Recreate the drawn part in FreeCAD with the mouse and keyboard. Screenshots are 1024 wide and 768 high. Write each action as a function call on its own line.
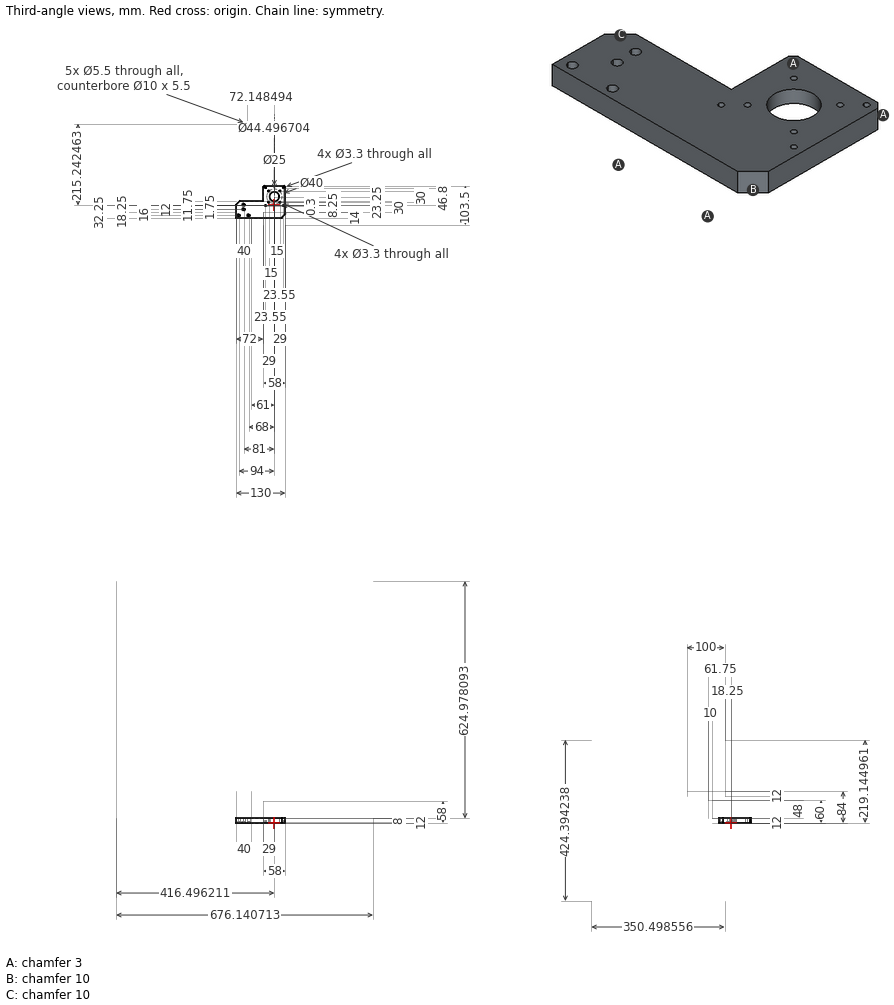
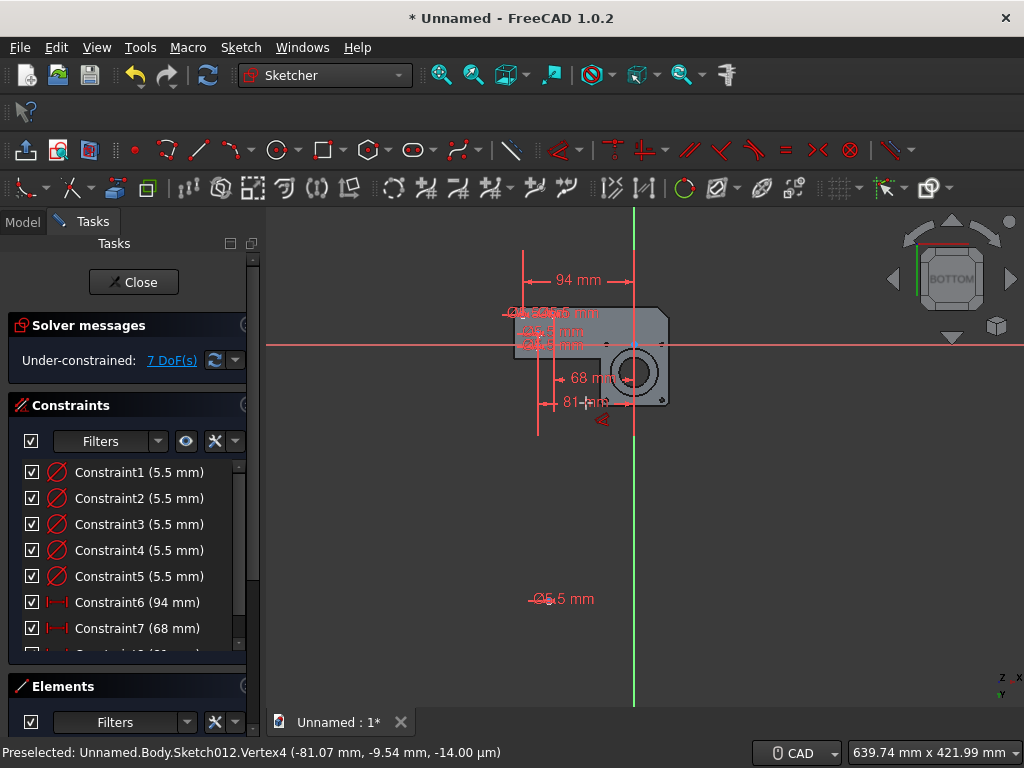
click(538, 347)
click(586, 311)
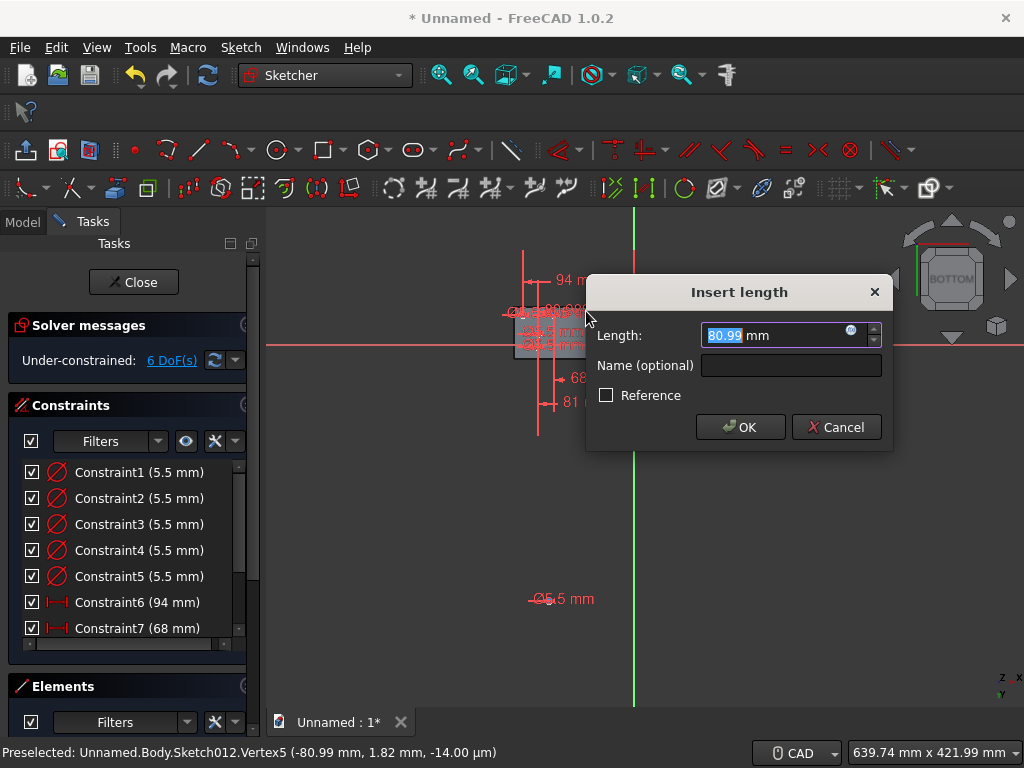
text(81)
key(Return)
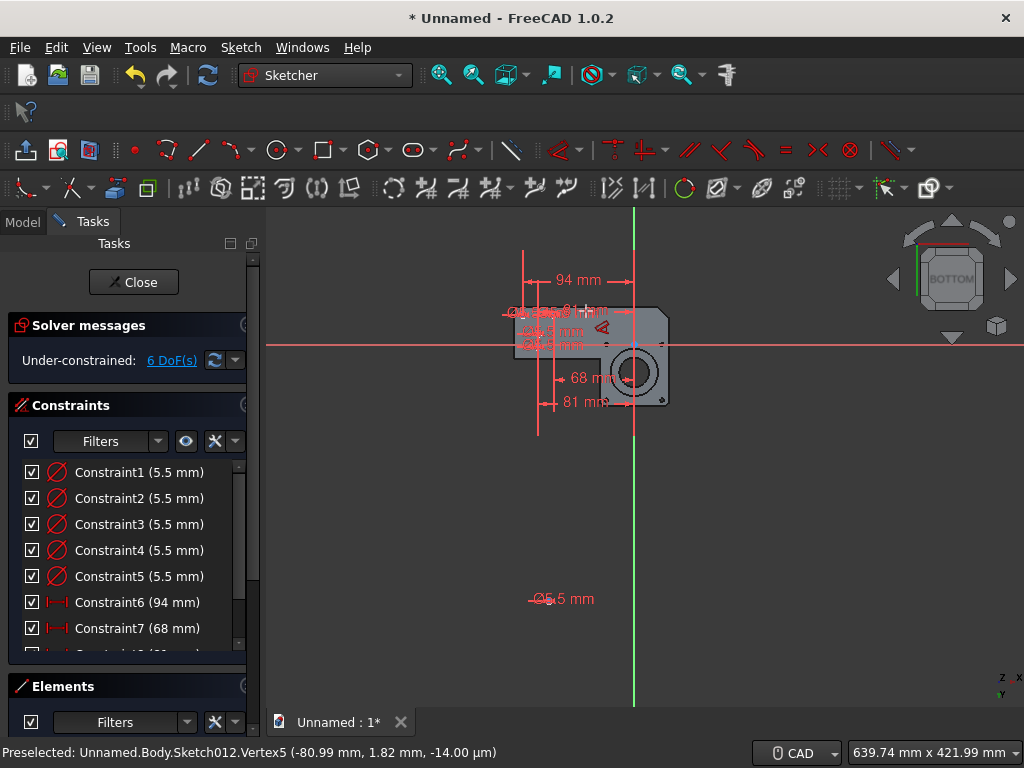
scroll(523, 315, up, 4)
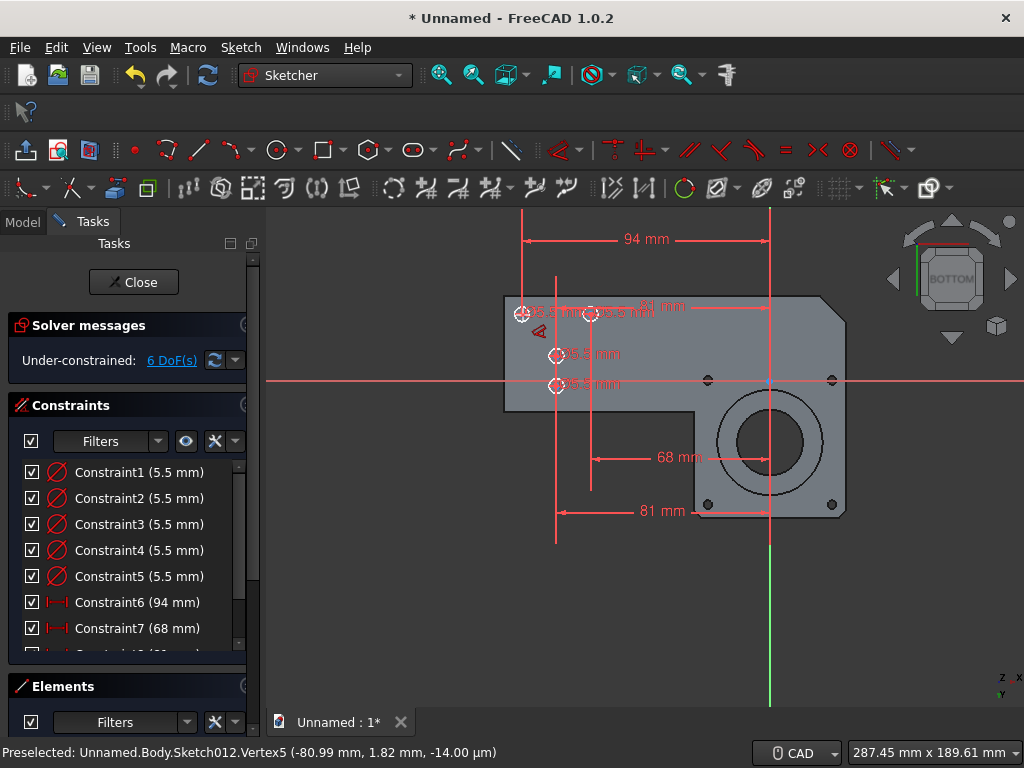
click(522, 314)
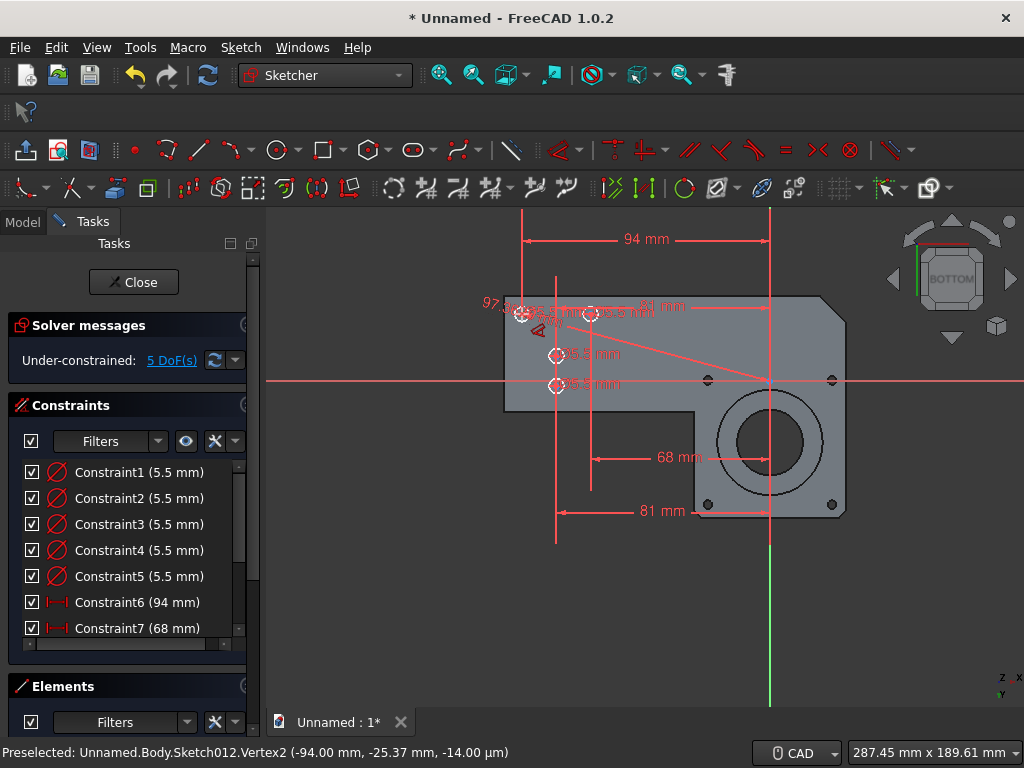
click(556, 356)
click(488, 335)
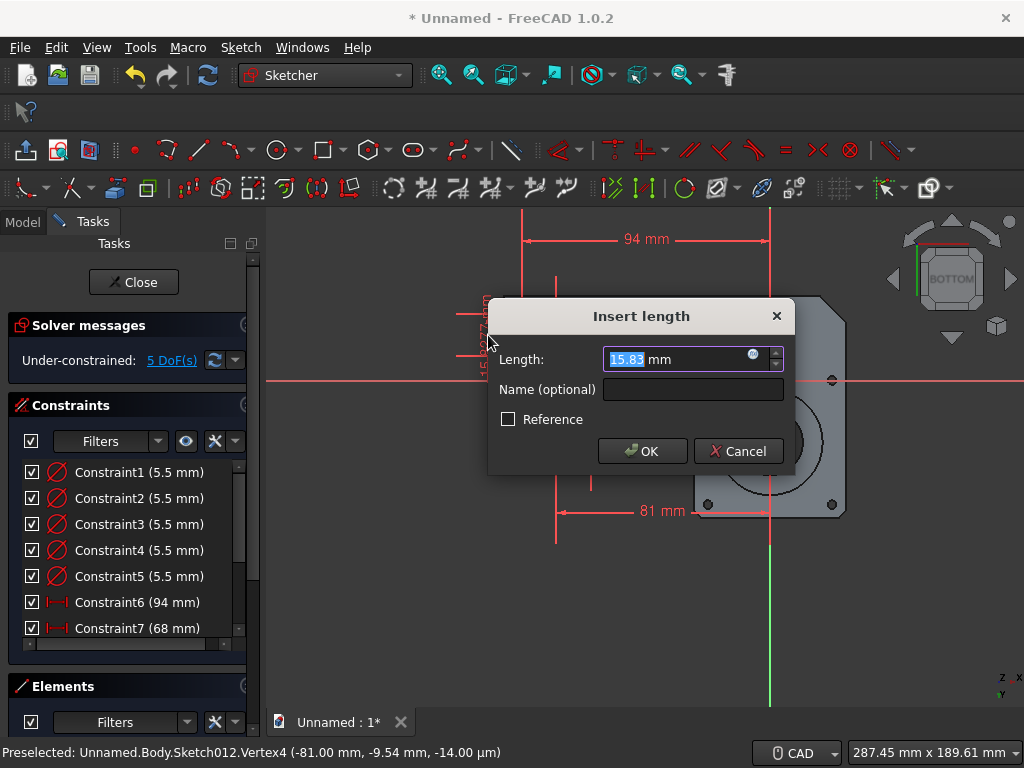
text(16)
key(Return)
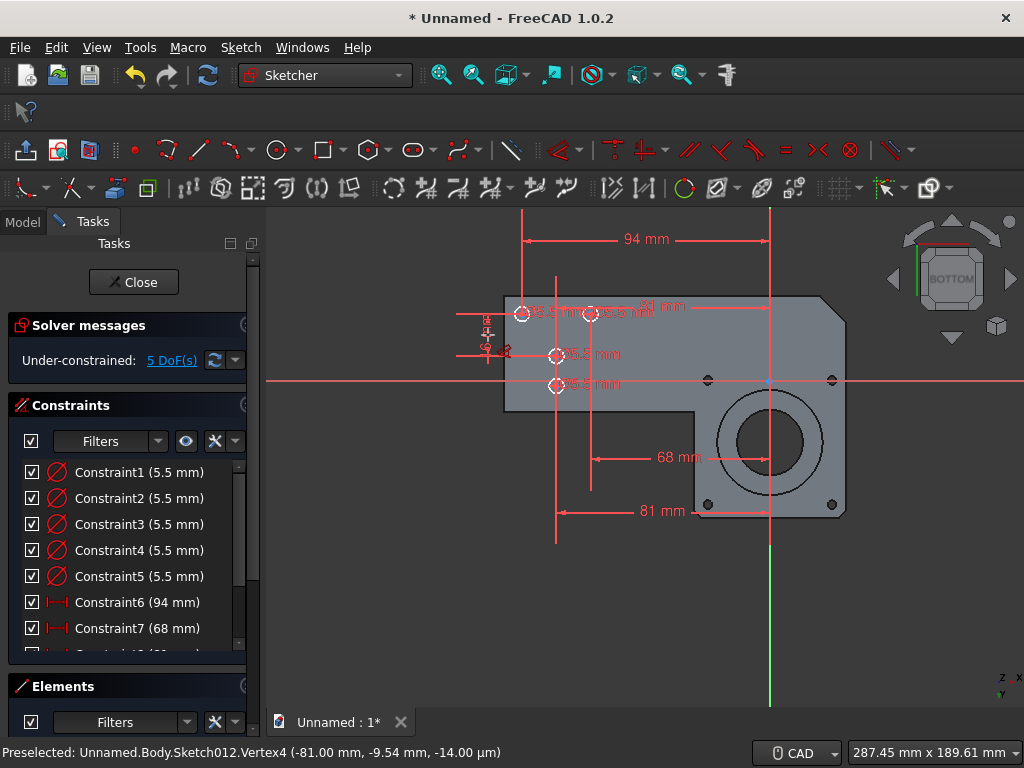
click(591, 314)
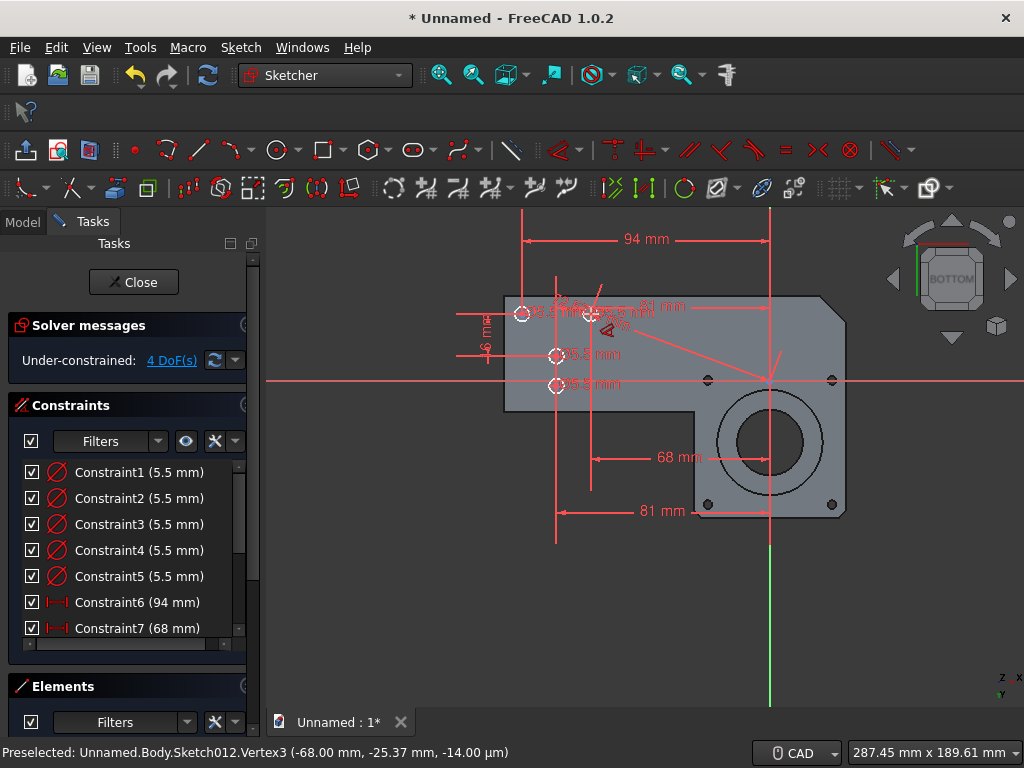
click(556, 356)
click(625, 335)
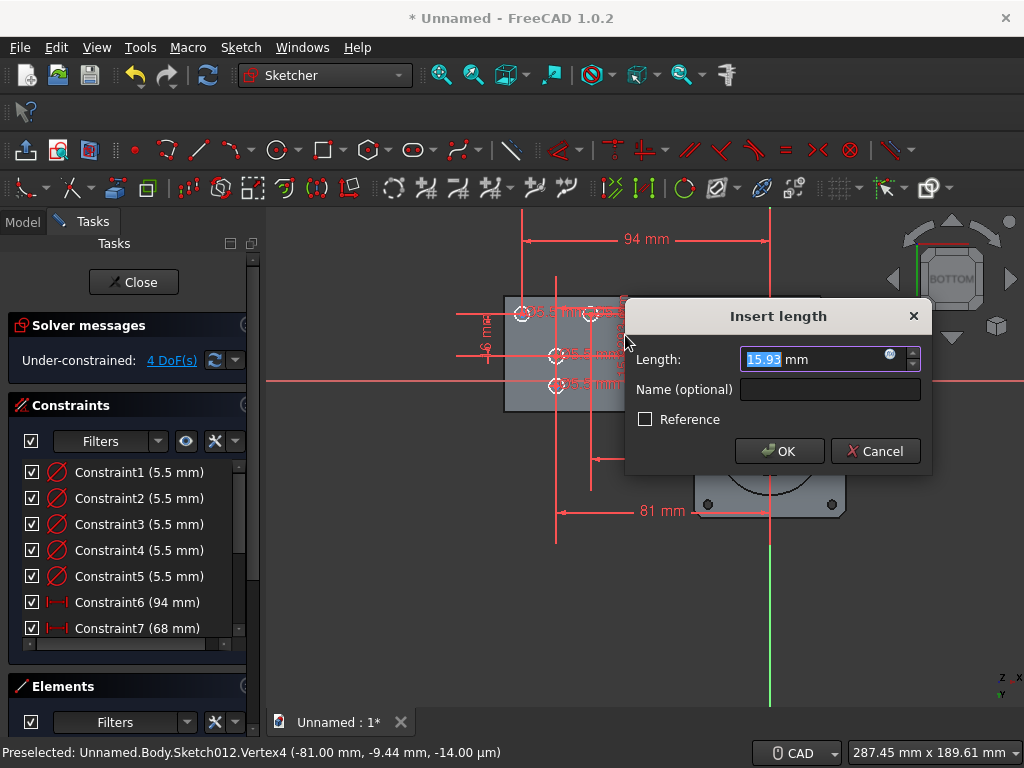
text(16)
key(Return)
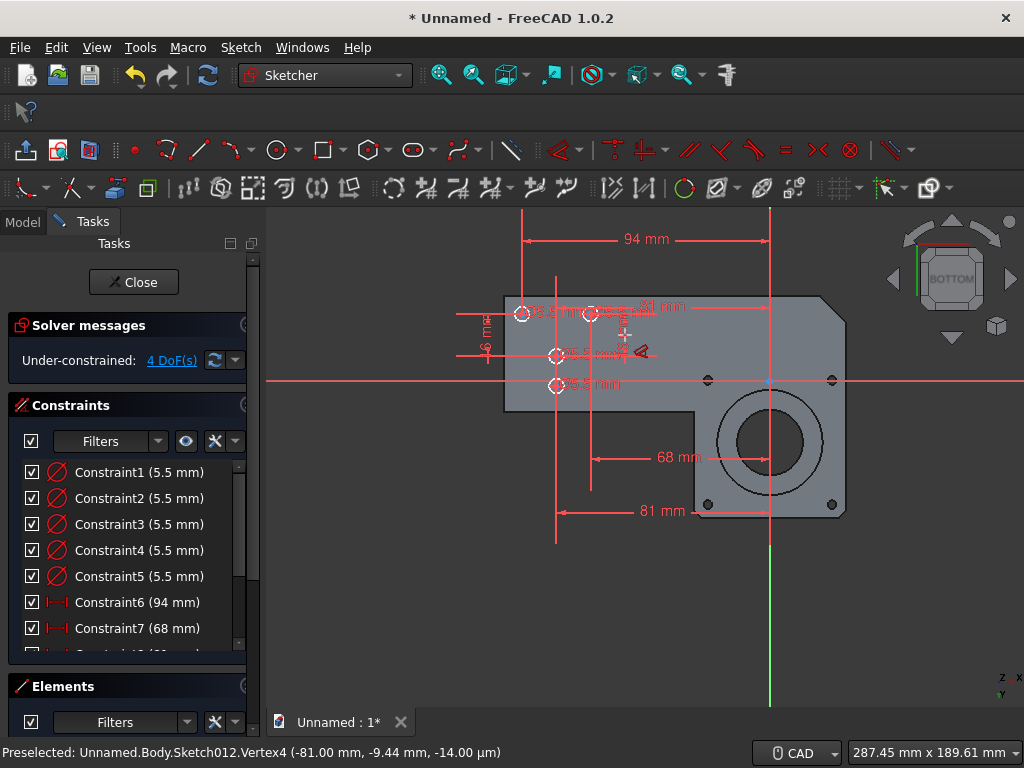
scroll(556, 356, up, 2)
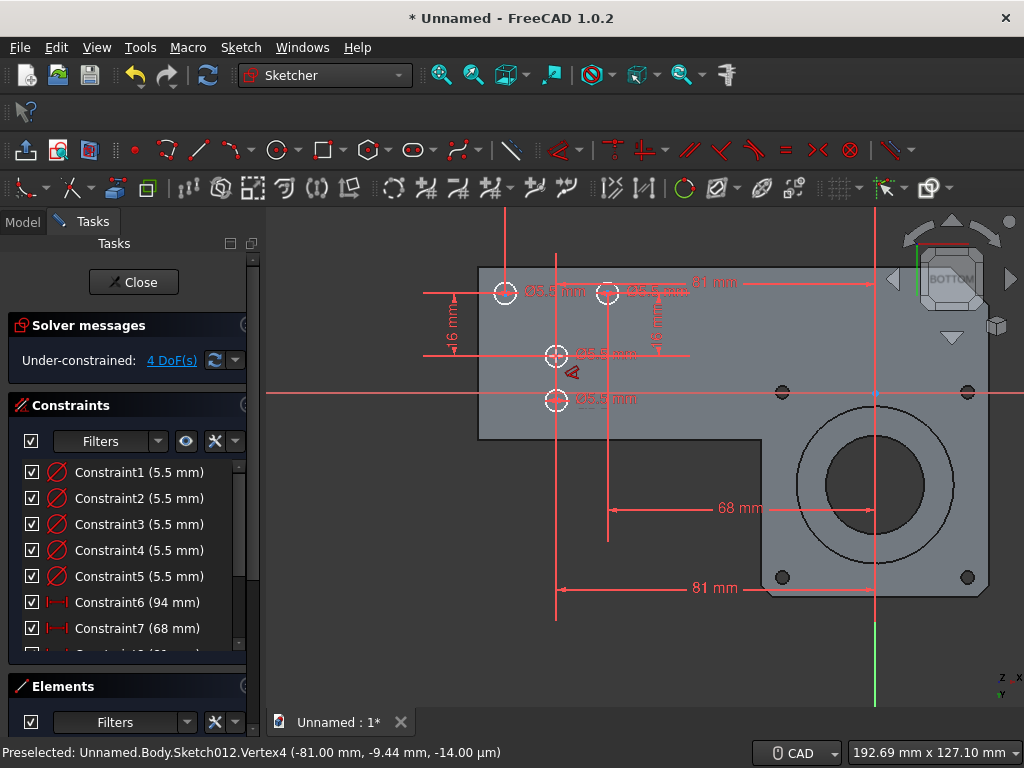
click(556, 356)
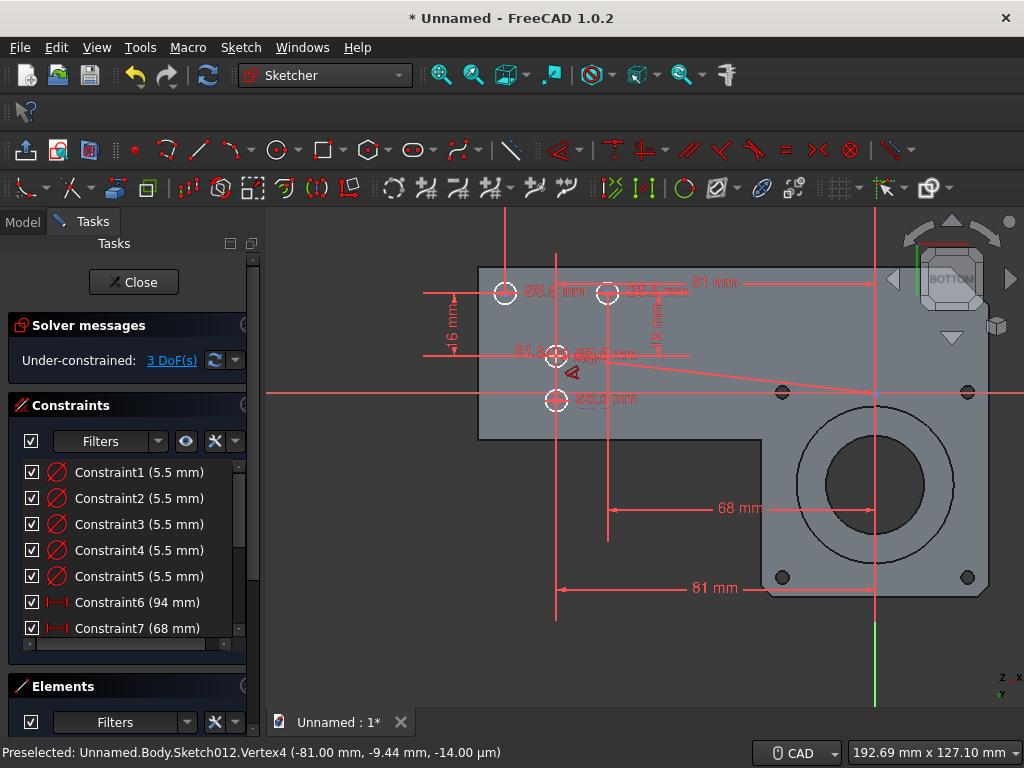
click(556, 401)
click(522, 378)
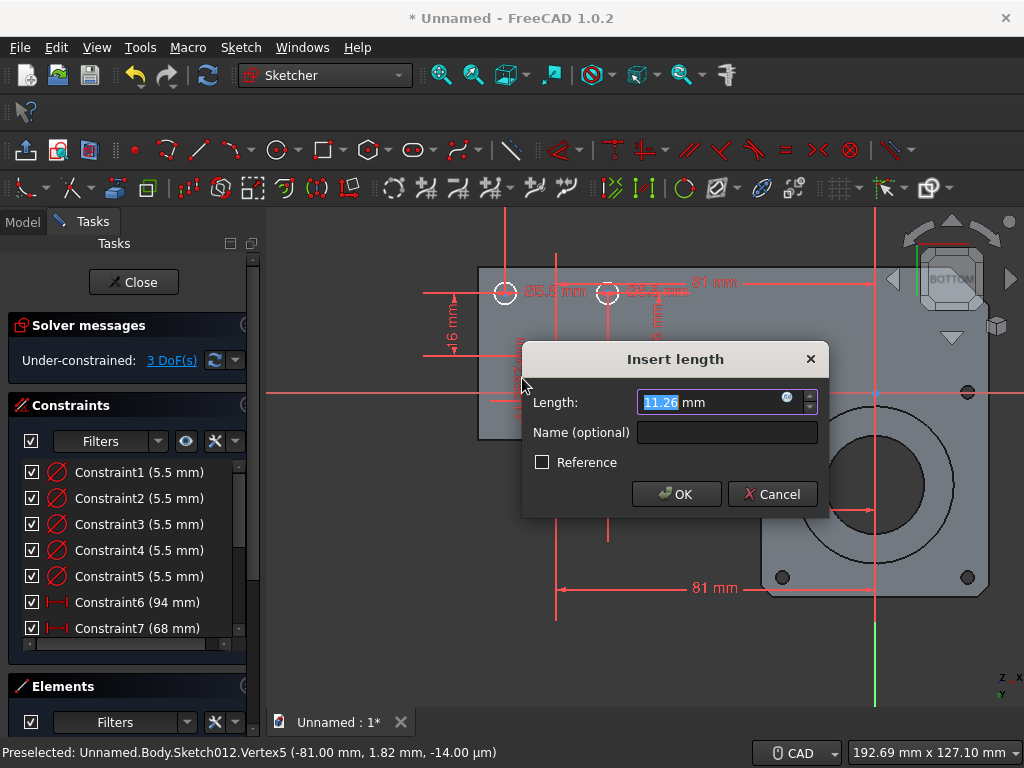
text(12)
key(Return)